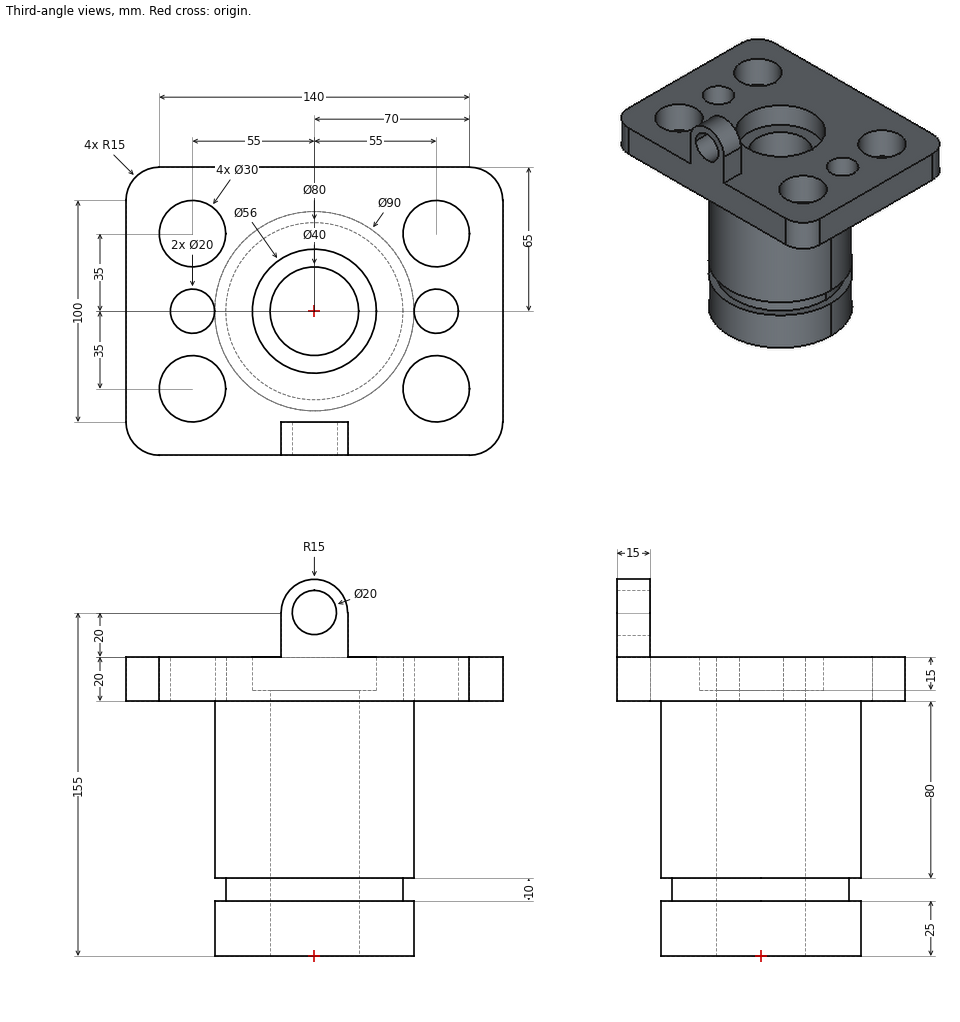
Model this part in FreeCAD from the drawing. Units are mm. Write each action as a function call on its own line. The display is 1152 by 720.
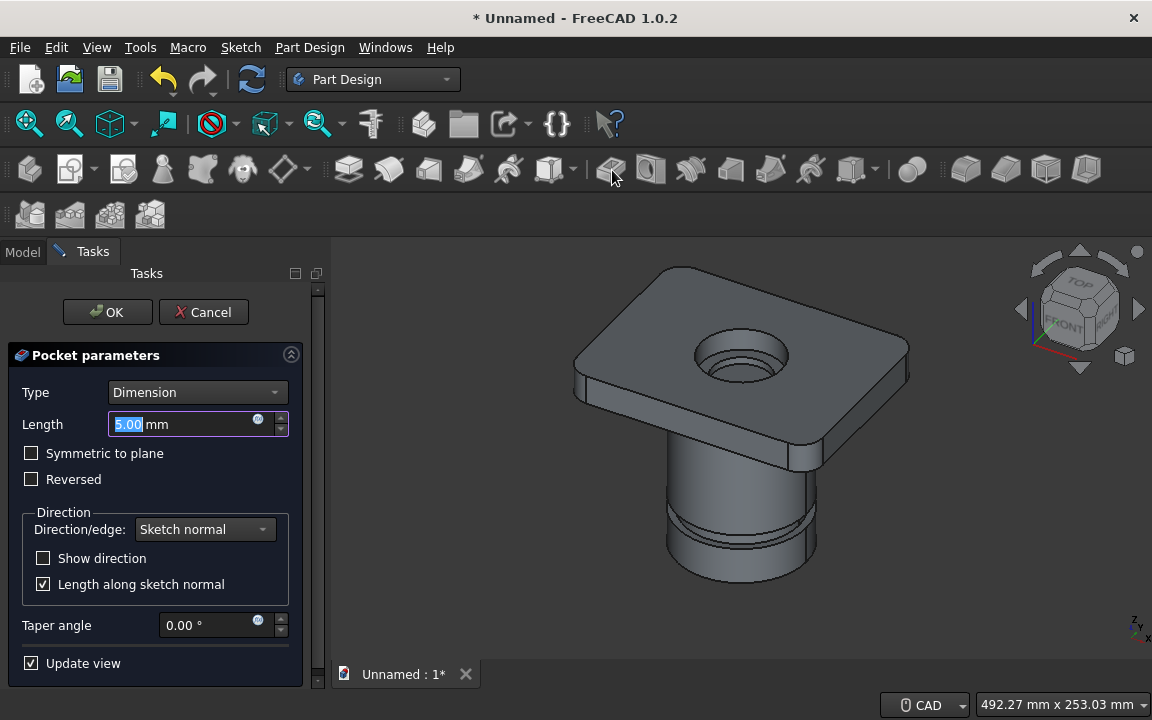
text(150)
key(Tab)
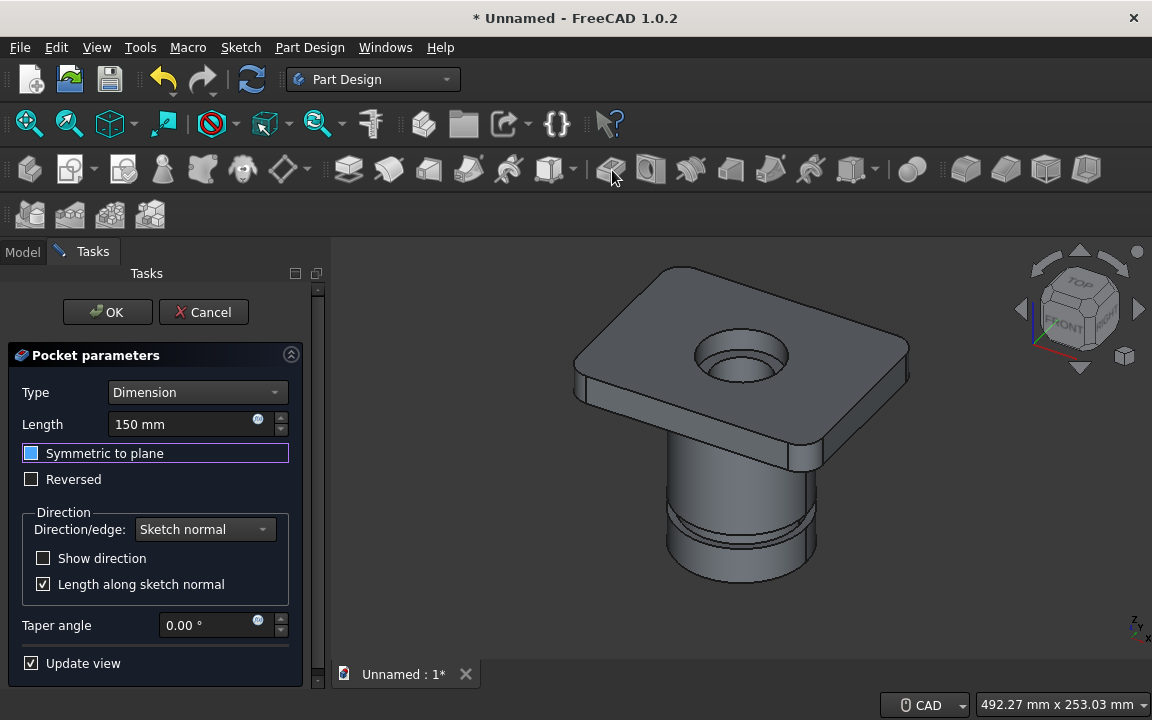
click(108, 312)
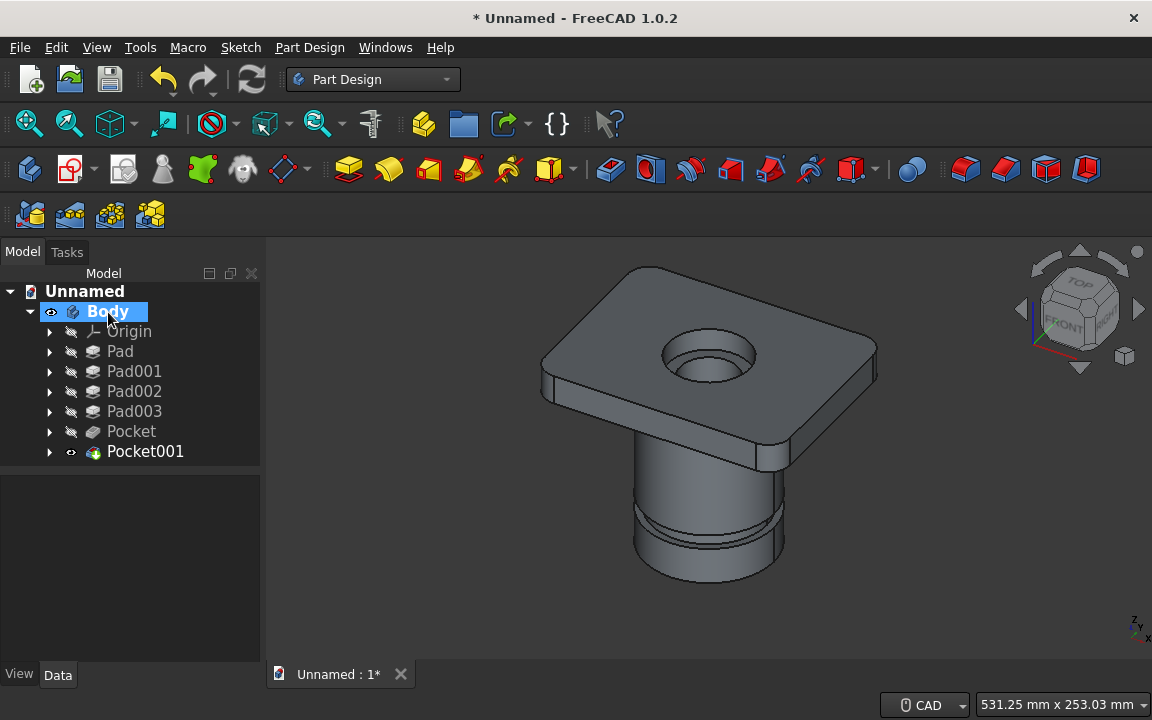
click(810, 347)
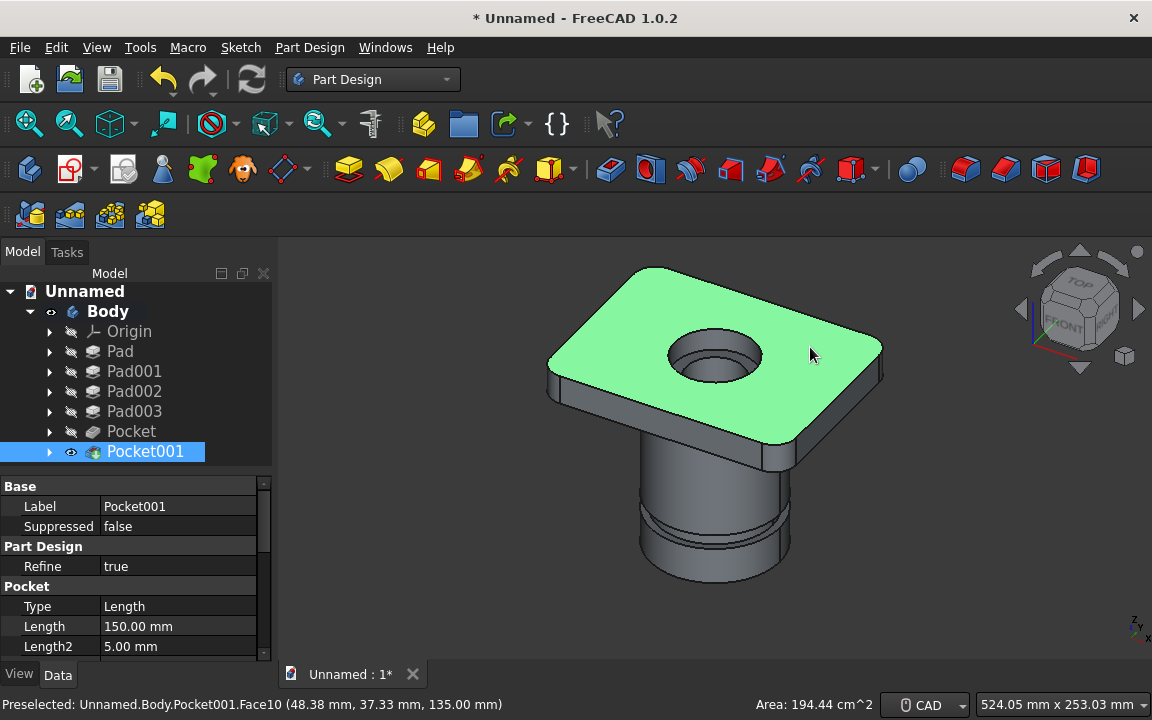
click(70, 170)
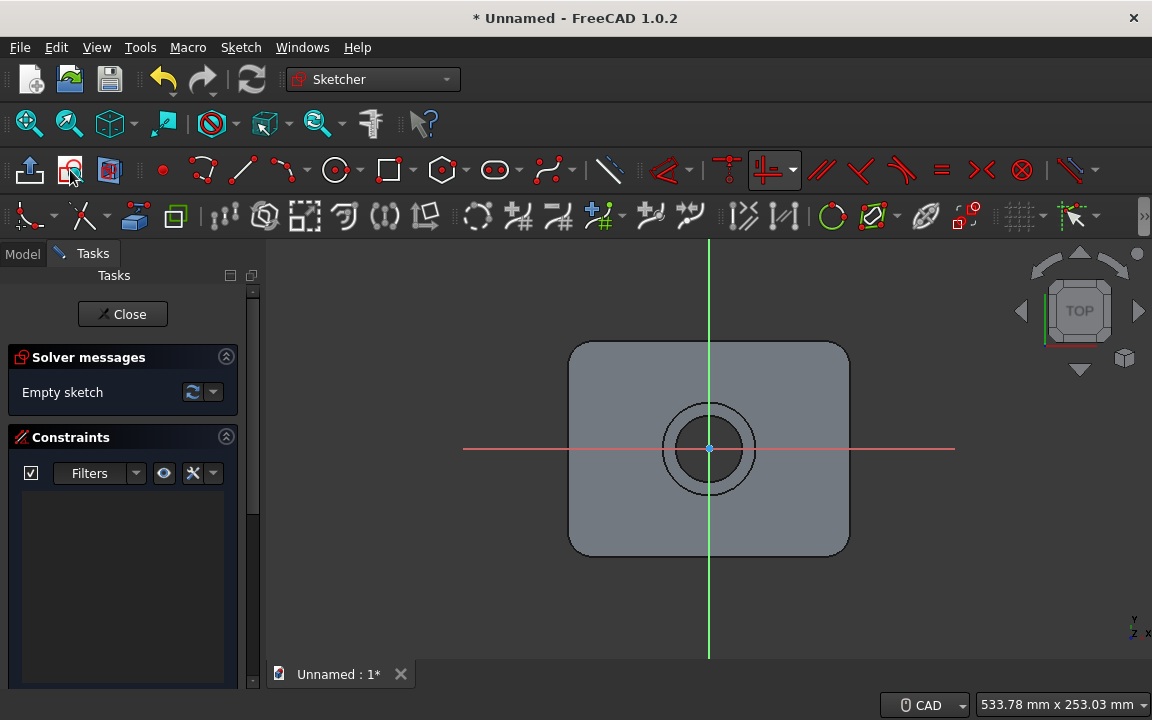
scroll(848, 449, up, 2)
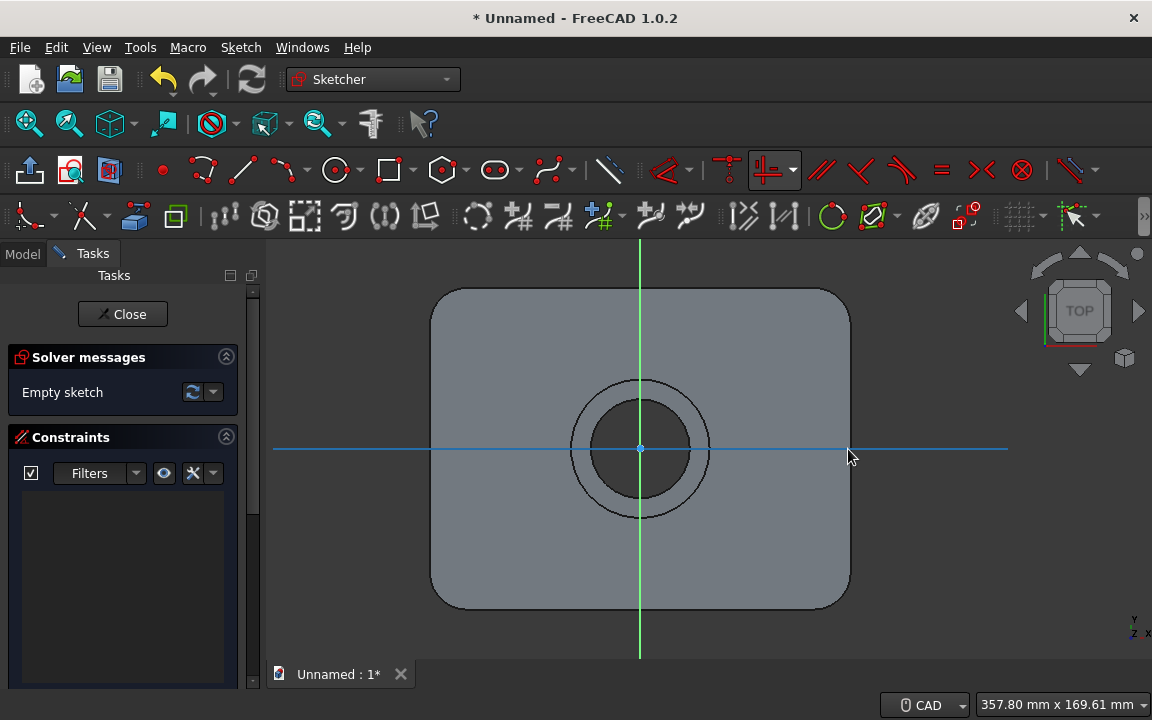
click(336, 170)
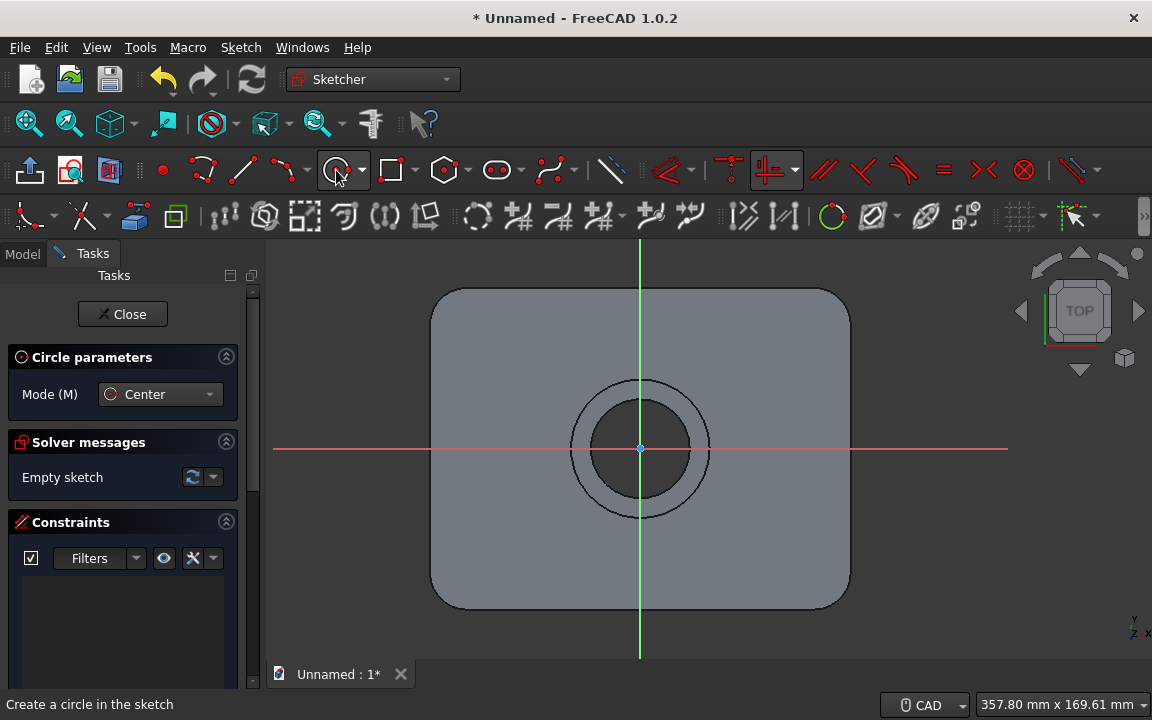
click(504, 362)
click(530, 336)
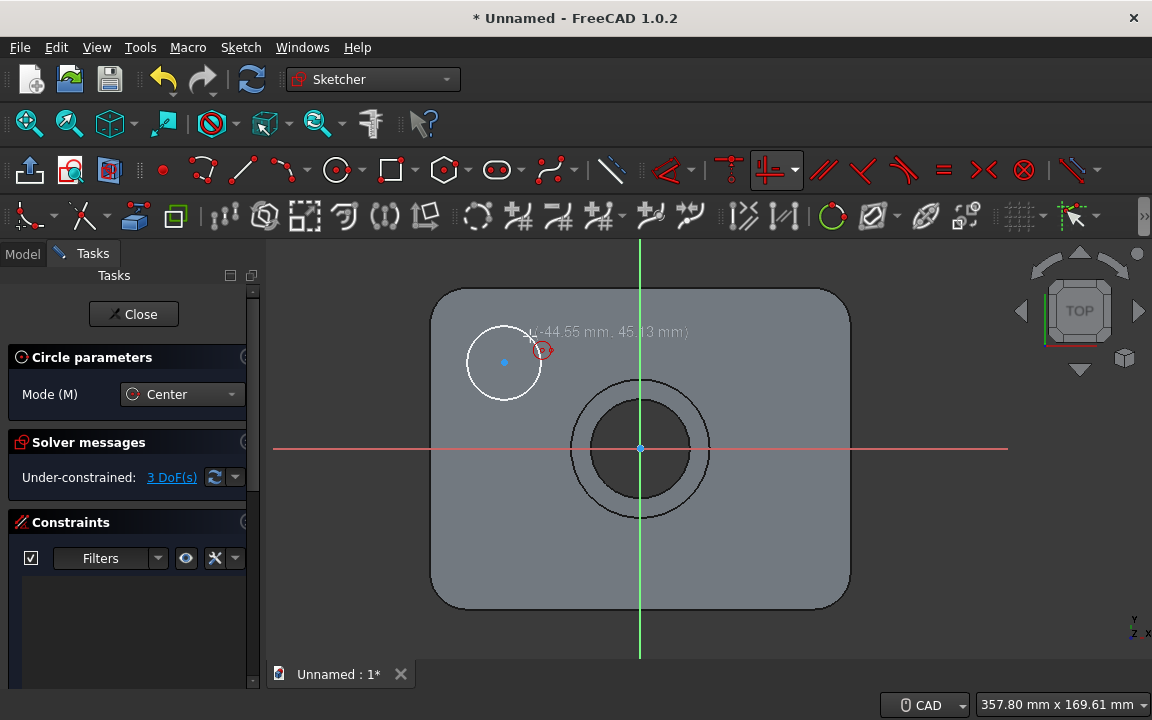
click(777, 362)
click(803, 336)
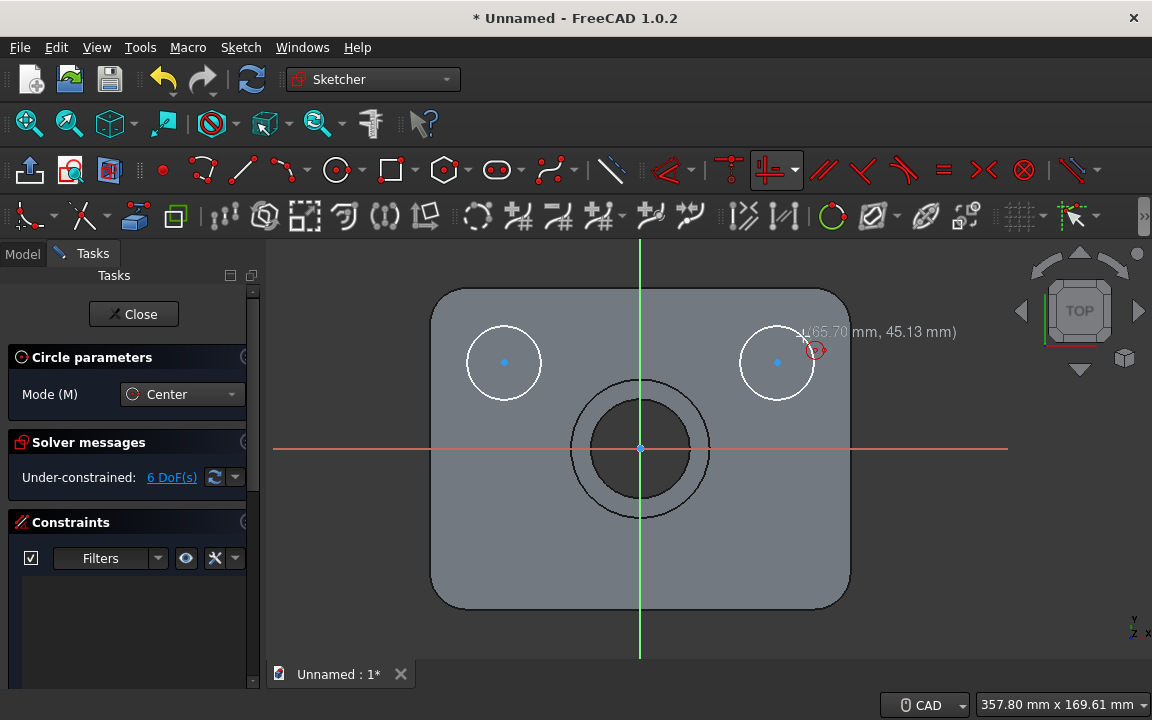
click(504, 535)
click(530, 509)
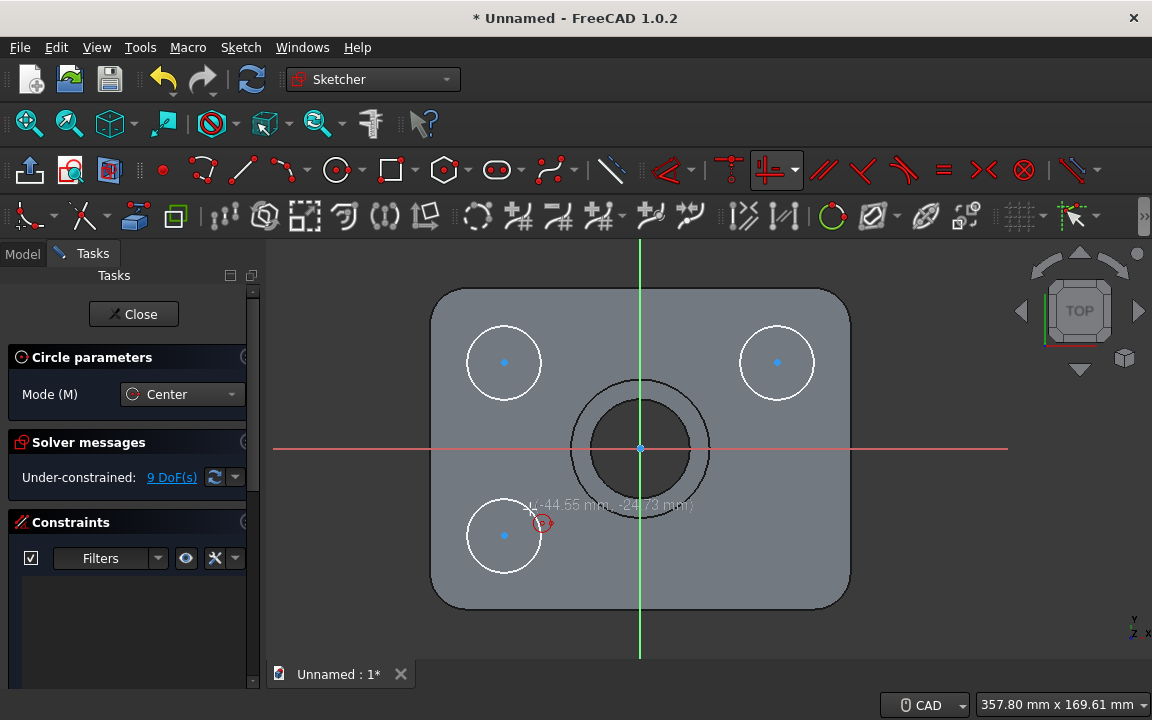
click(777, 535)
click(803, 509)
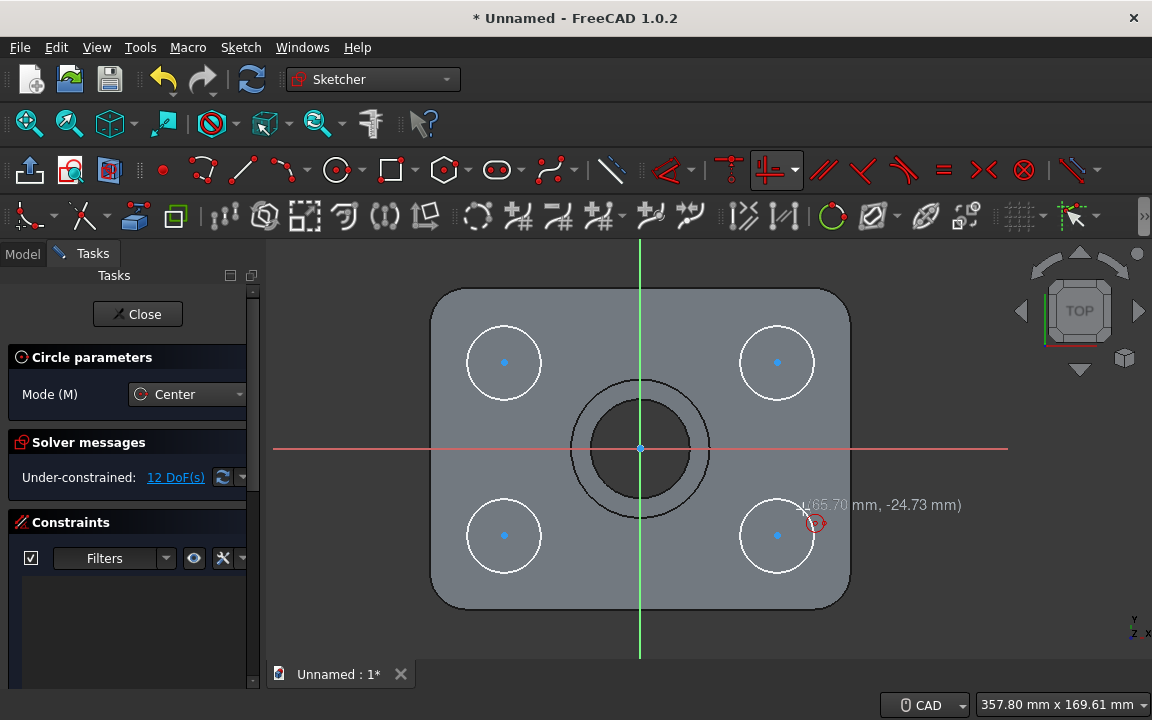
click(504, 449)
click(522, 431)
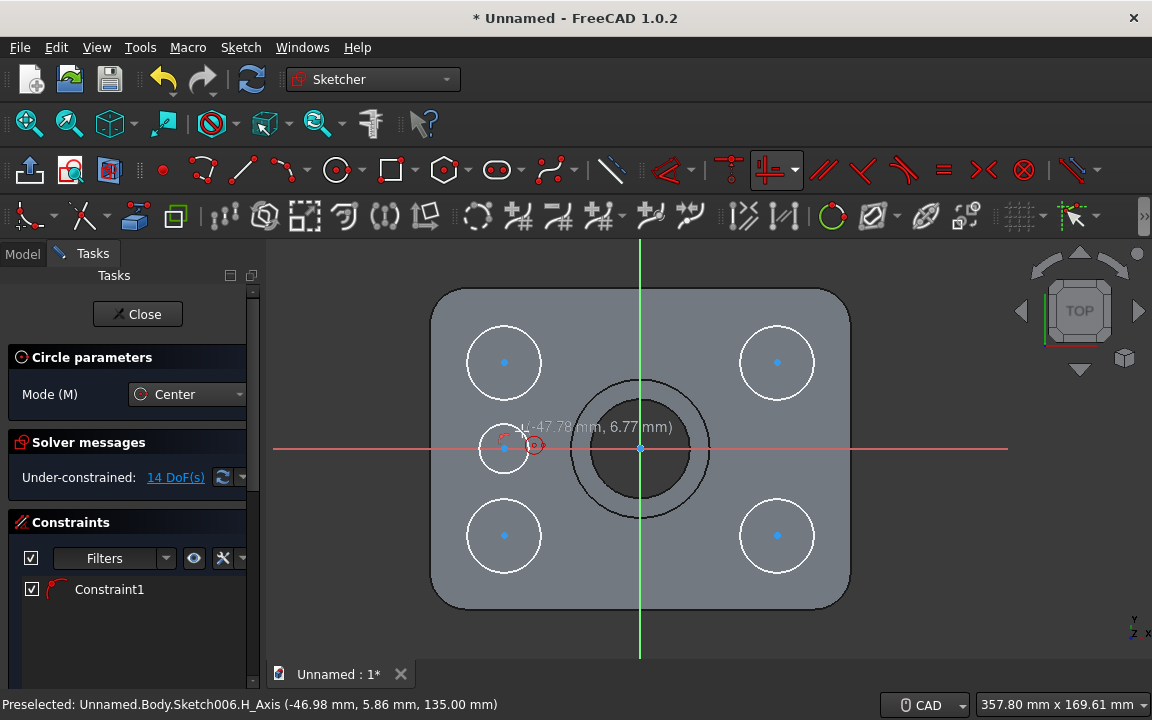
click(777, 449)
click(794, 431)
key(Escape)